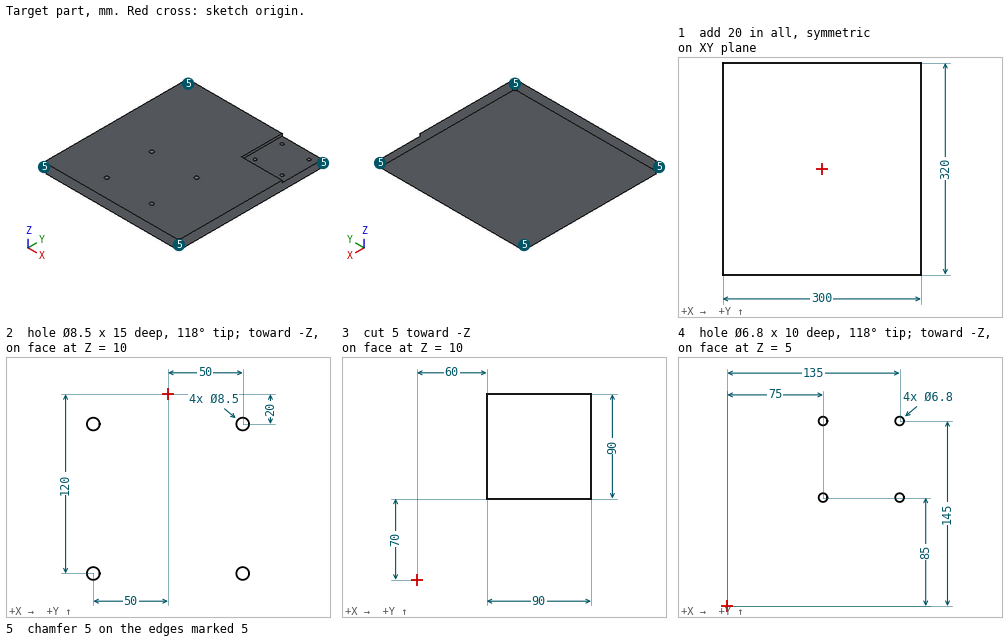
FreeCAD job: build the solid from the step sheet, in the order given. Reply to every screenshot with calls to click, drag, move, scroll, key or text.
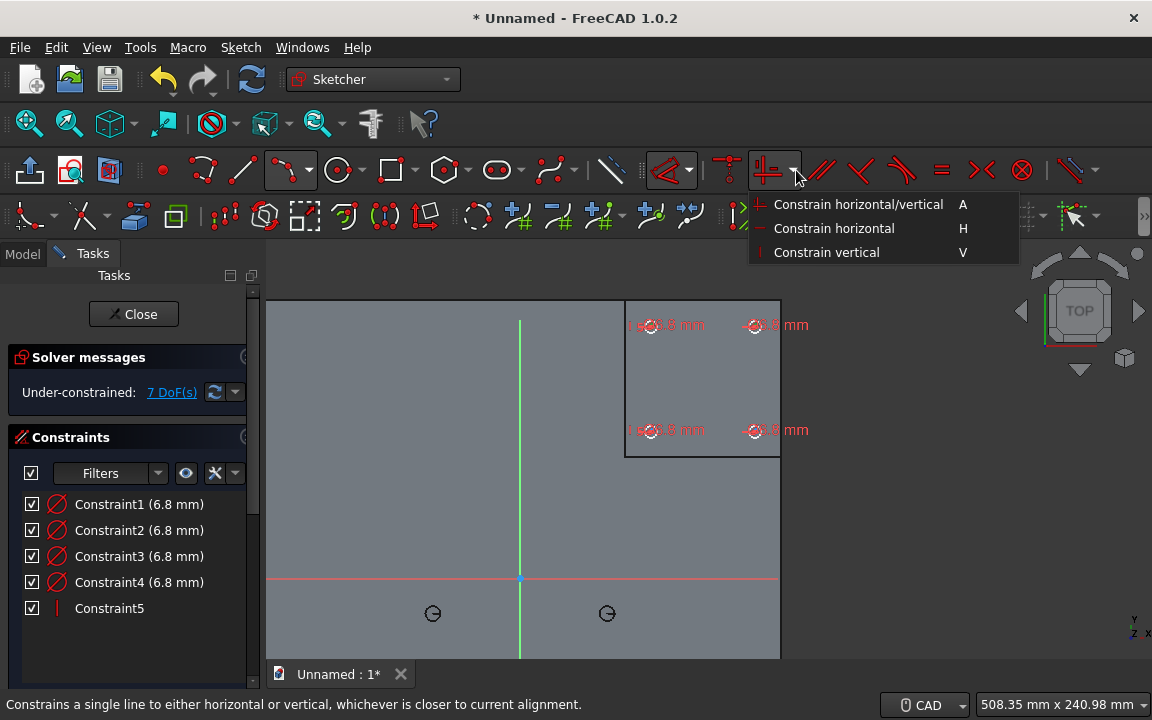
click(884, 228)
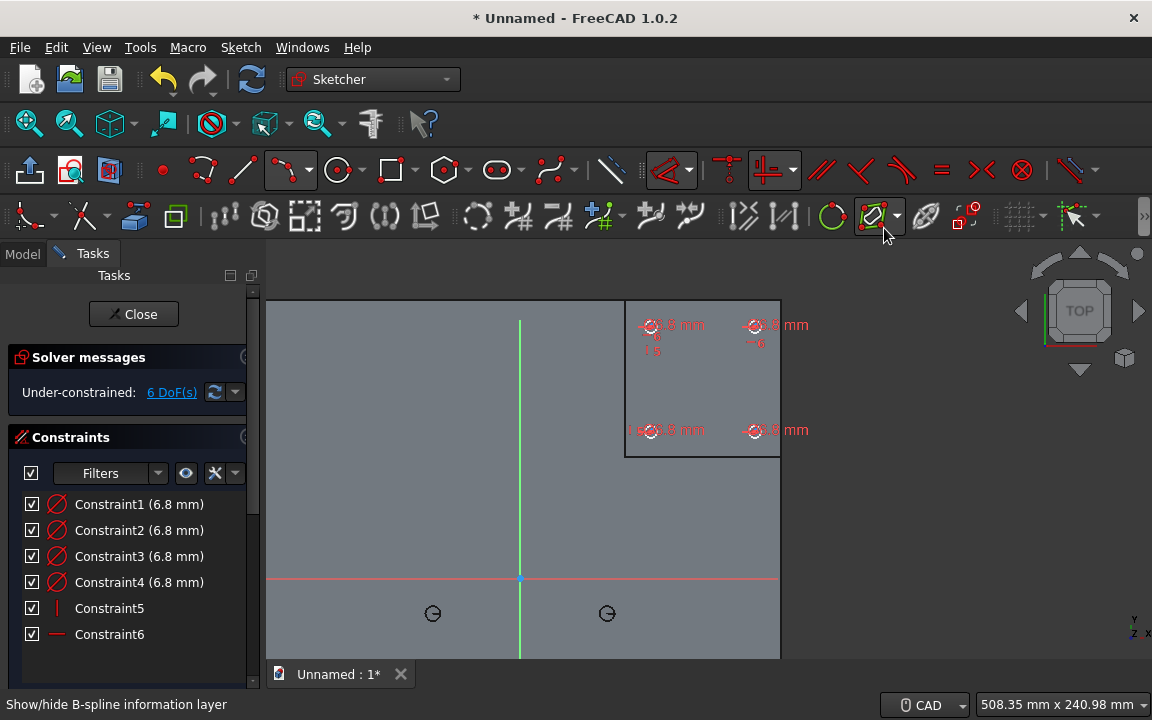
click(755, 327)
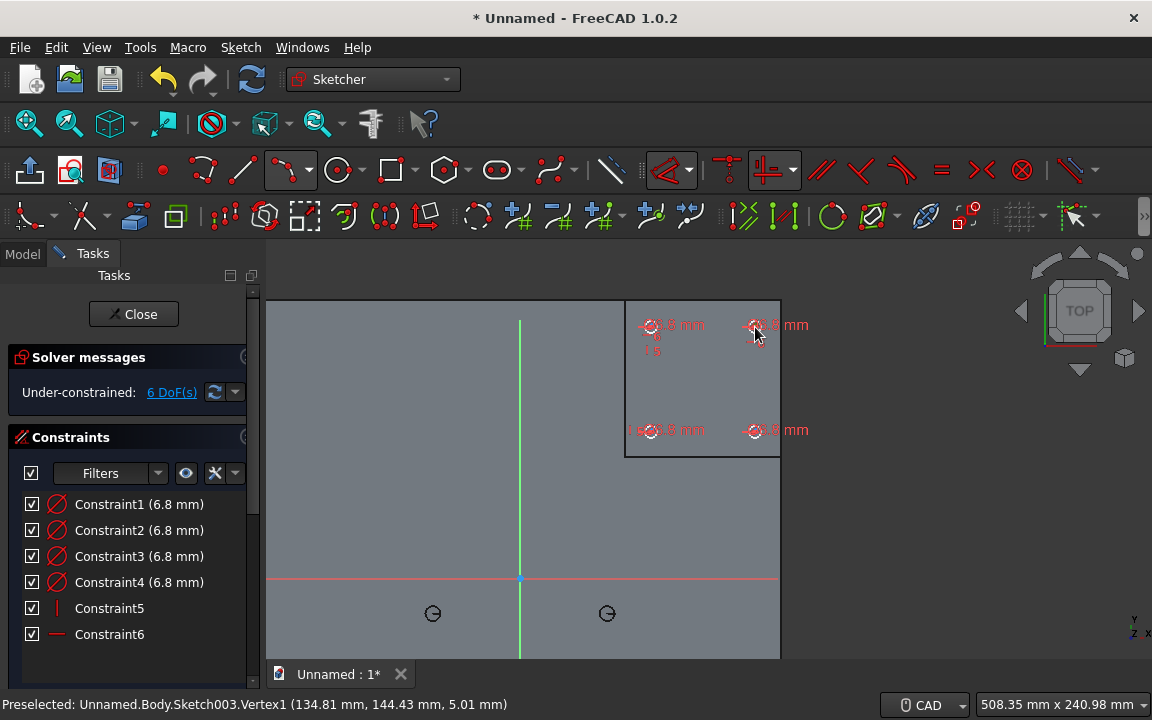
click(755, 432)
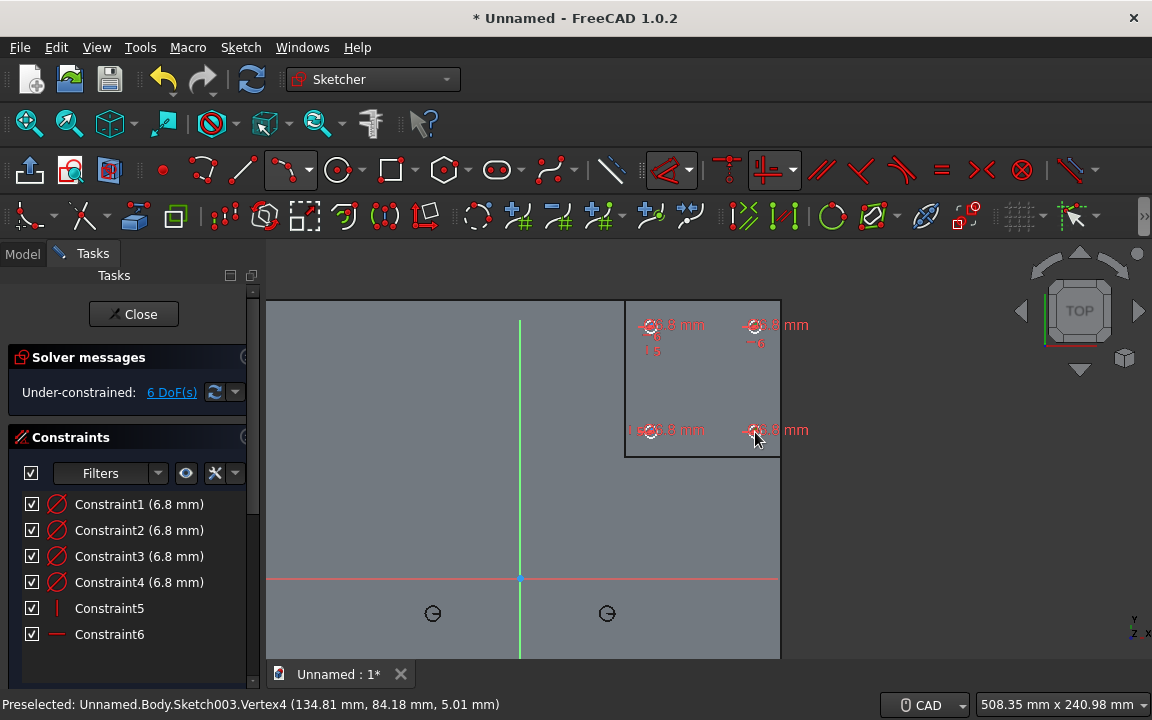
key(v)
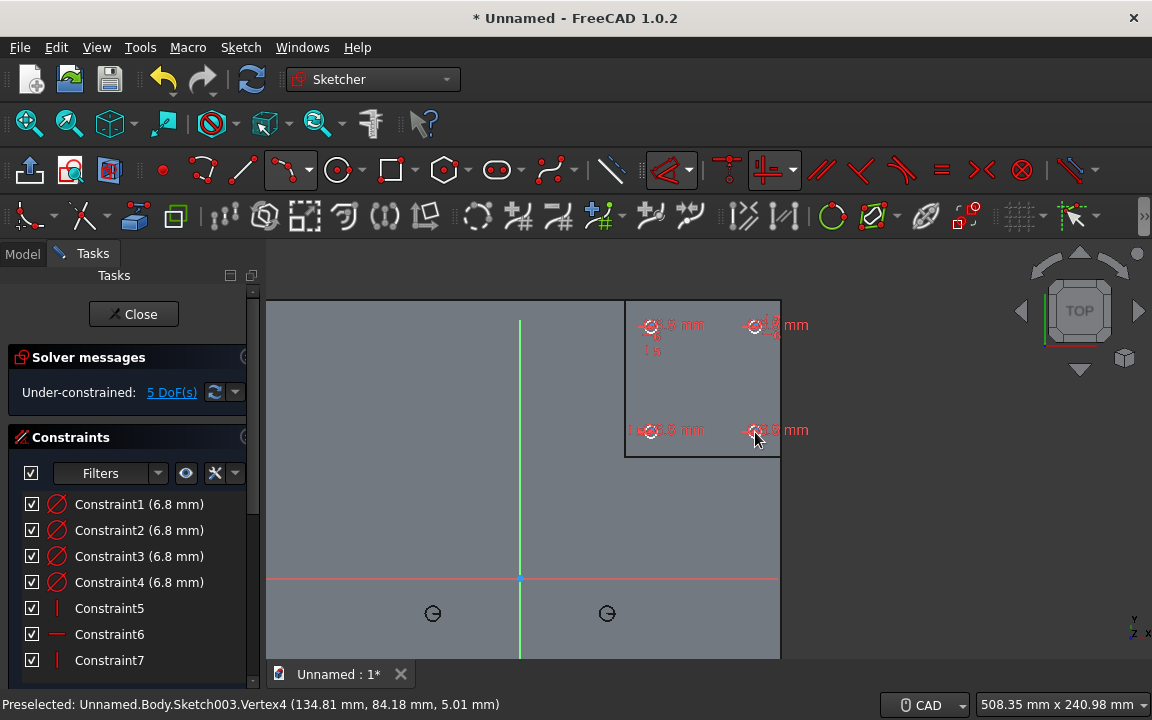
click(651, 432)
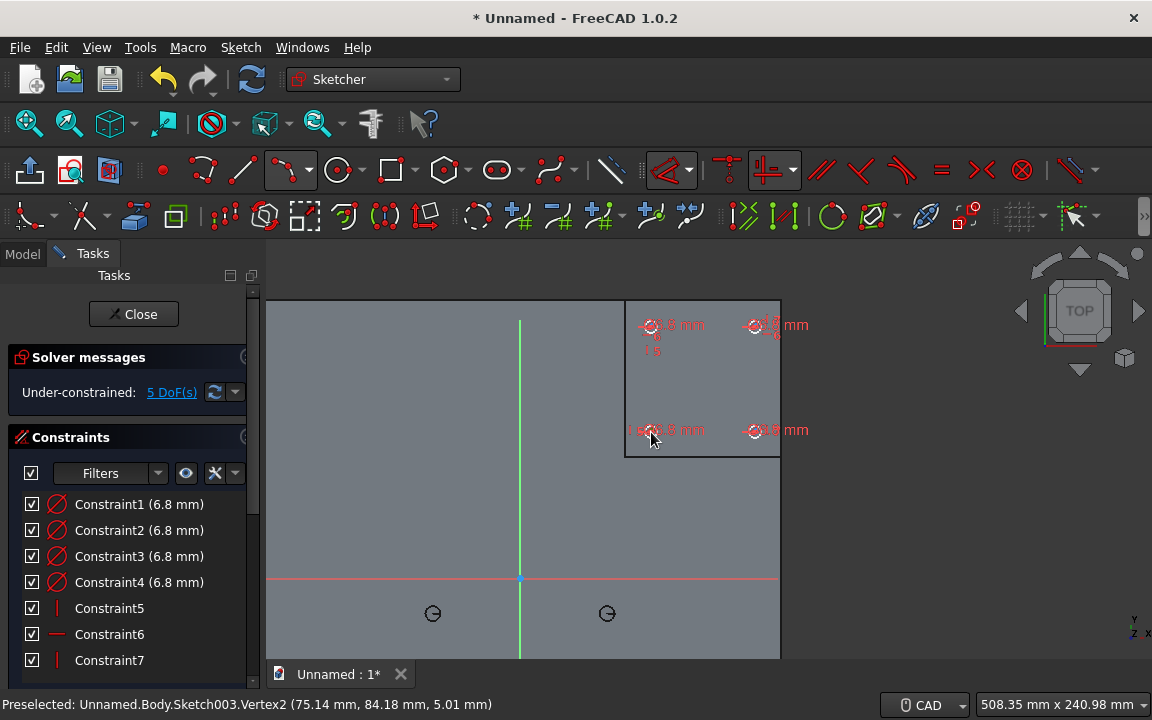
click(755, 432)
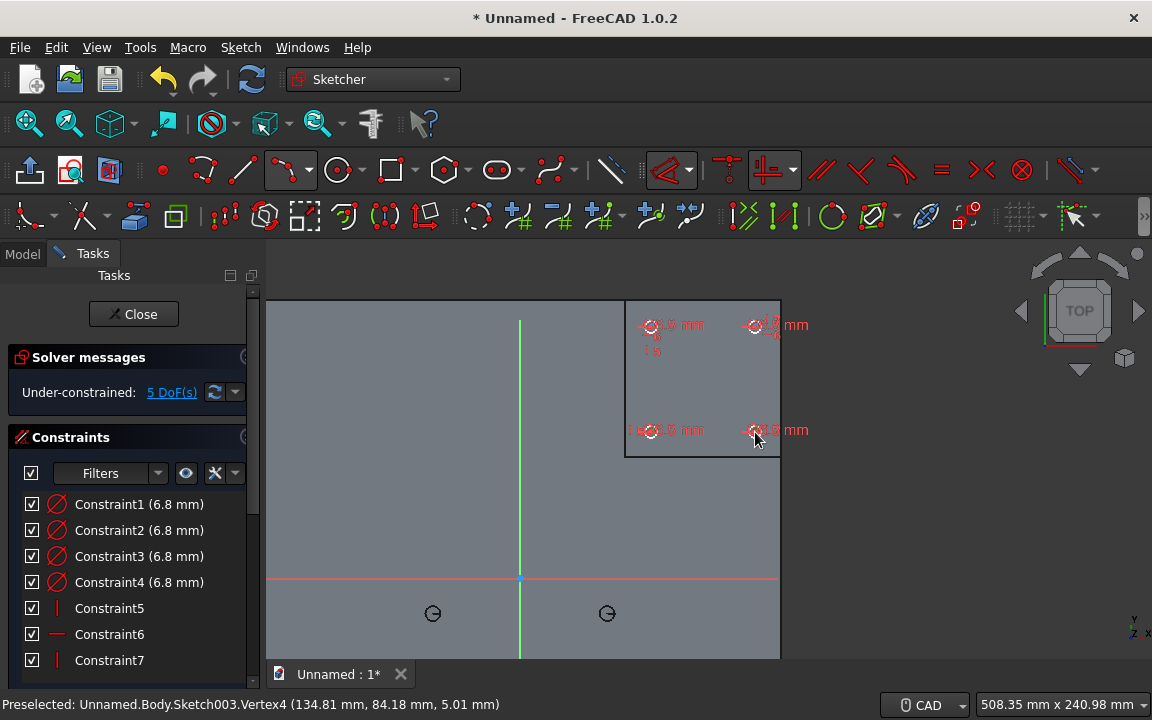
key(h)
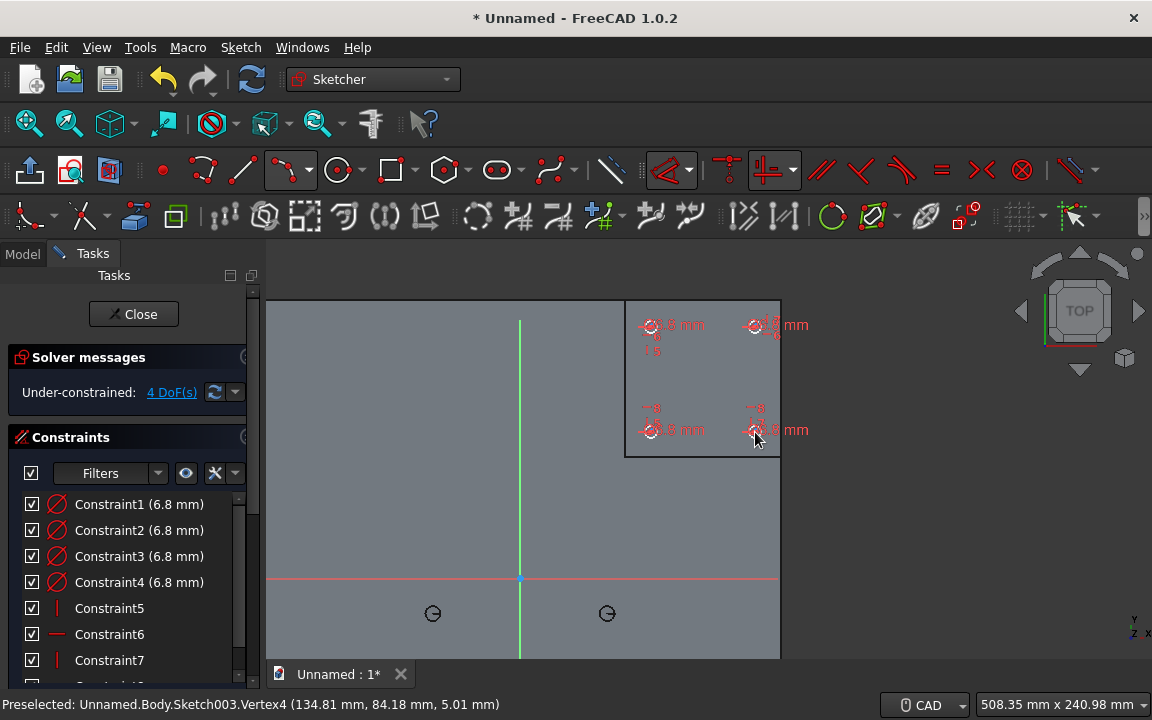
click(651, 432)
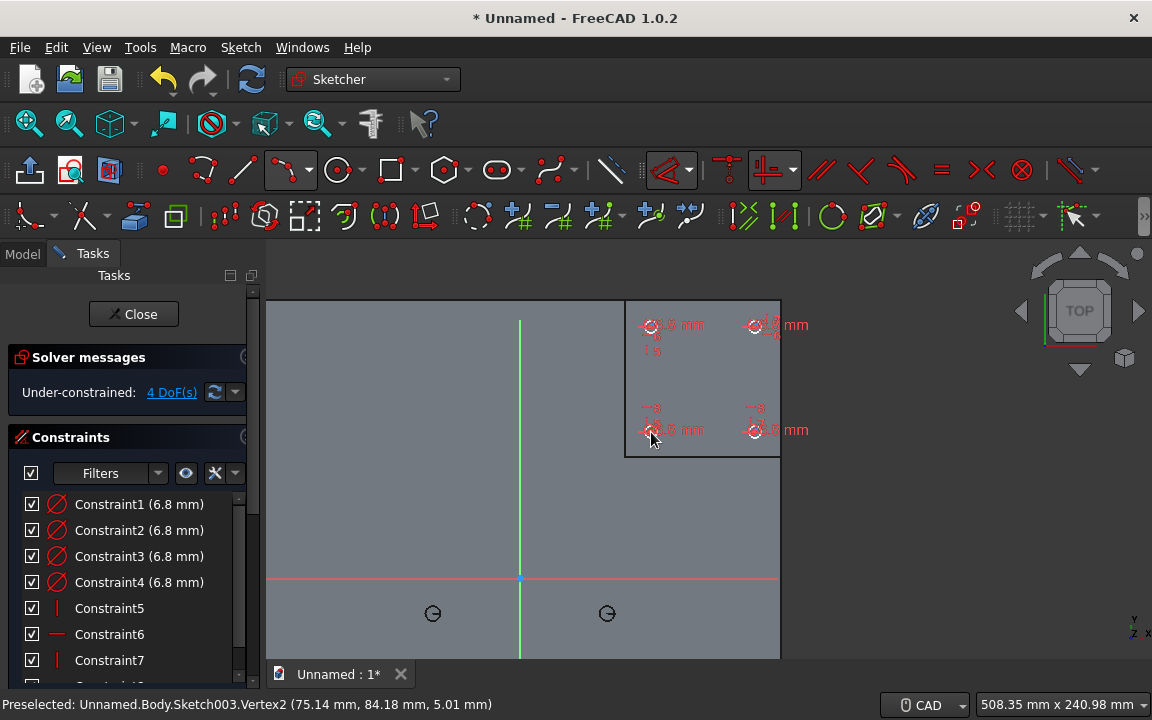
key(l)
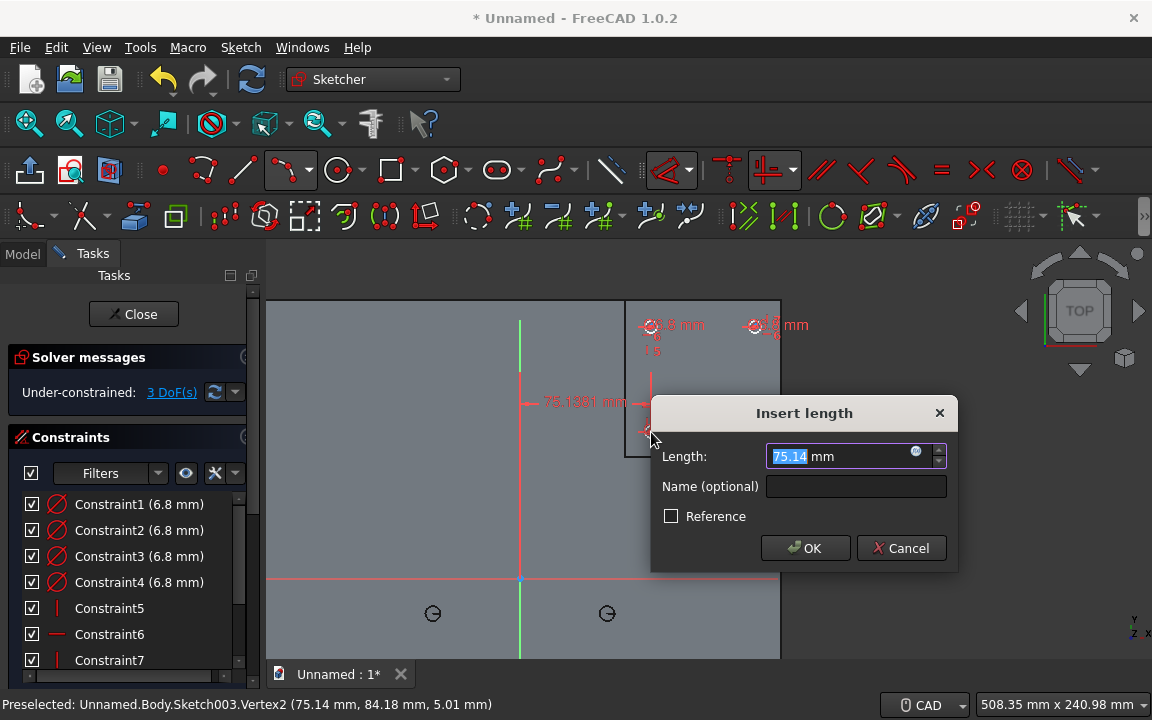
text(75)
key(Return)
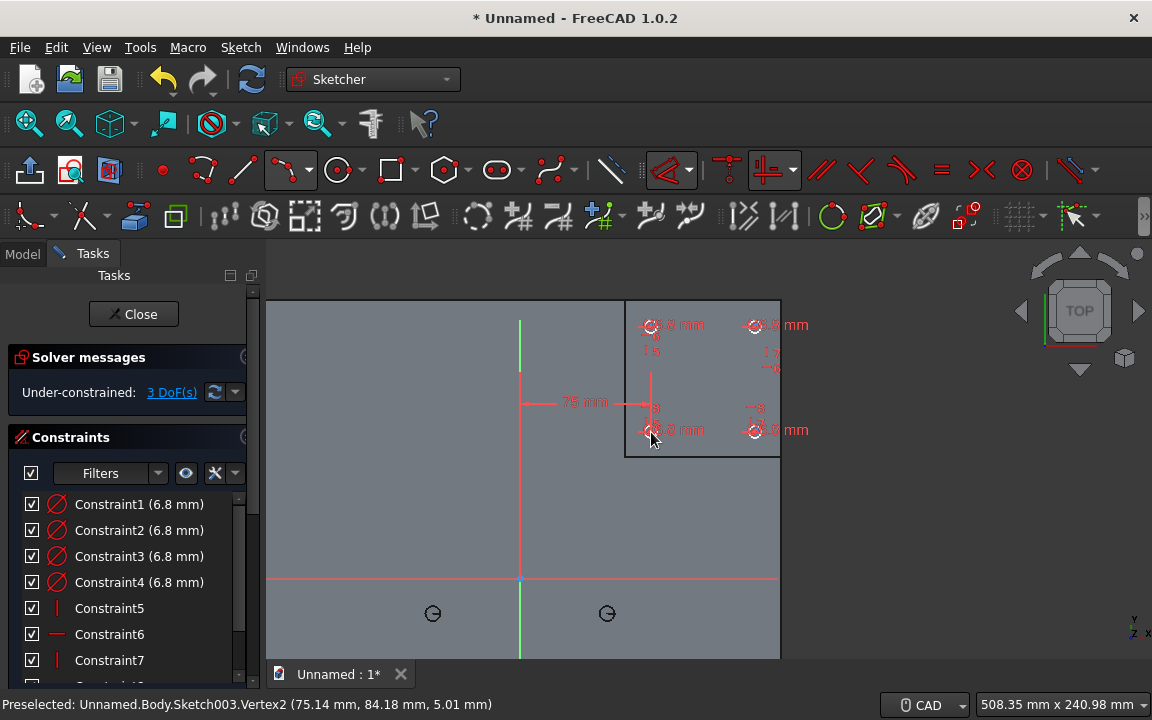
click(651, 432)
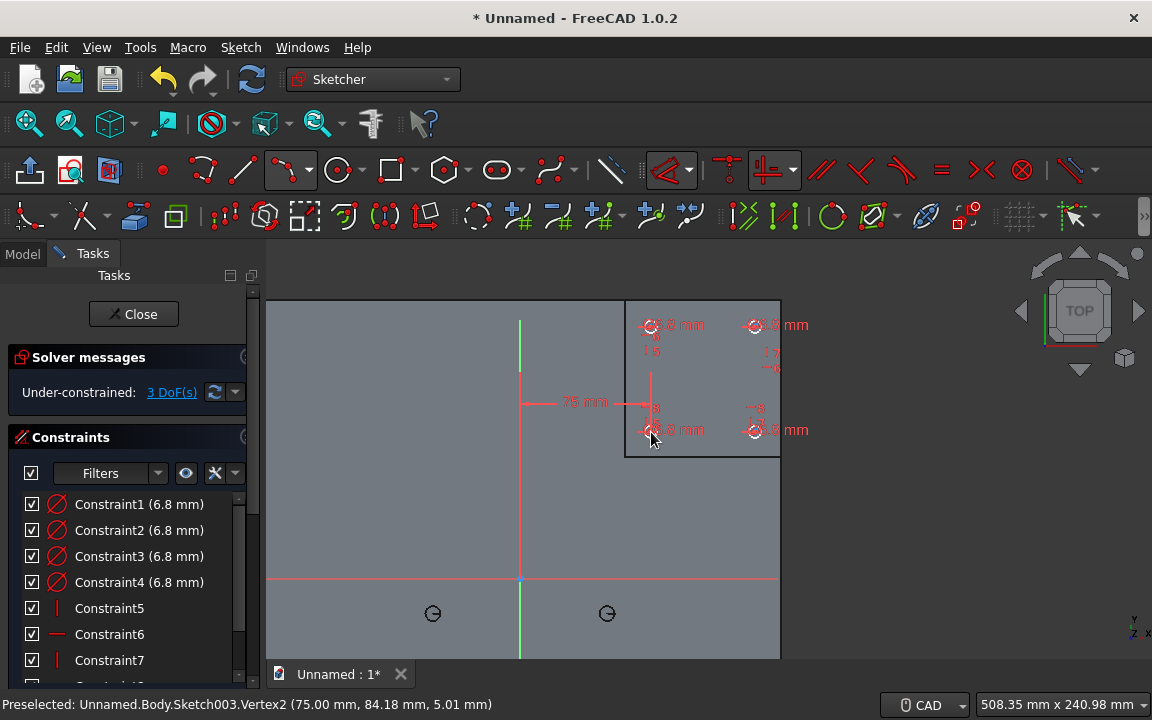
key(i)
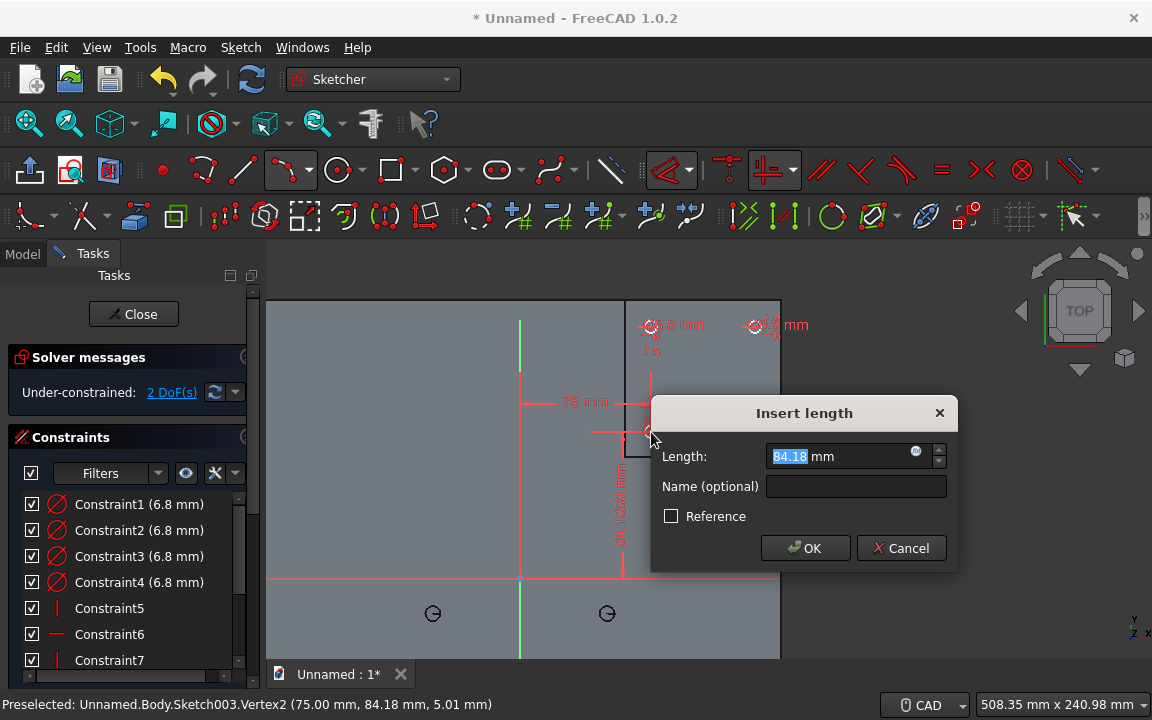
text(85)
key(Return)